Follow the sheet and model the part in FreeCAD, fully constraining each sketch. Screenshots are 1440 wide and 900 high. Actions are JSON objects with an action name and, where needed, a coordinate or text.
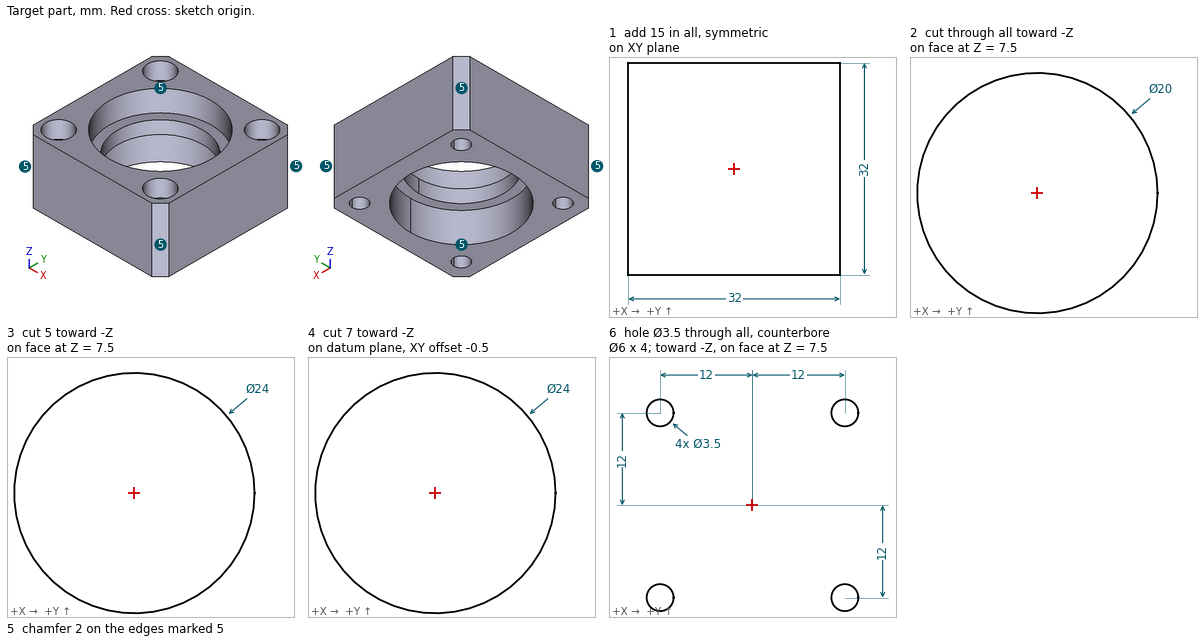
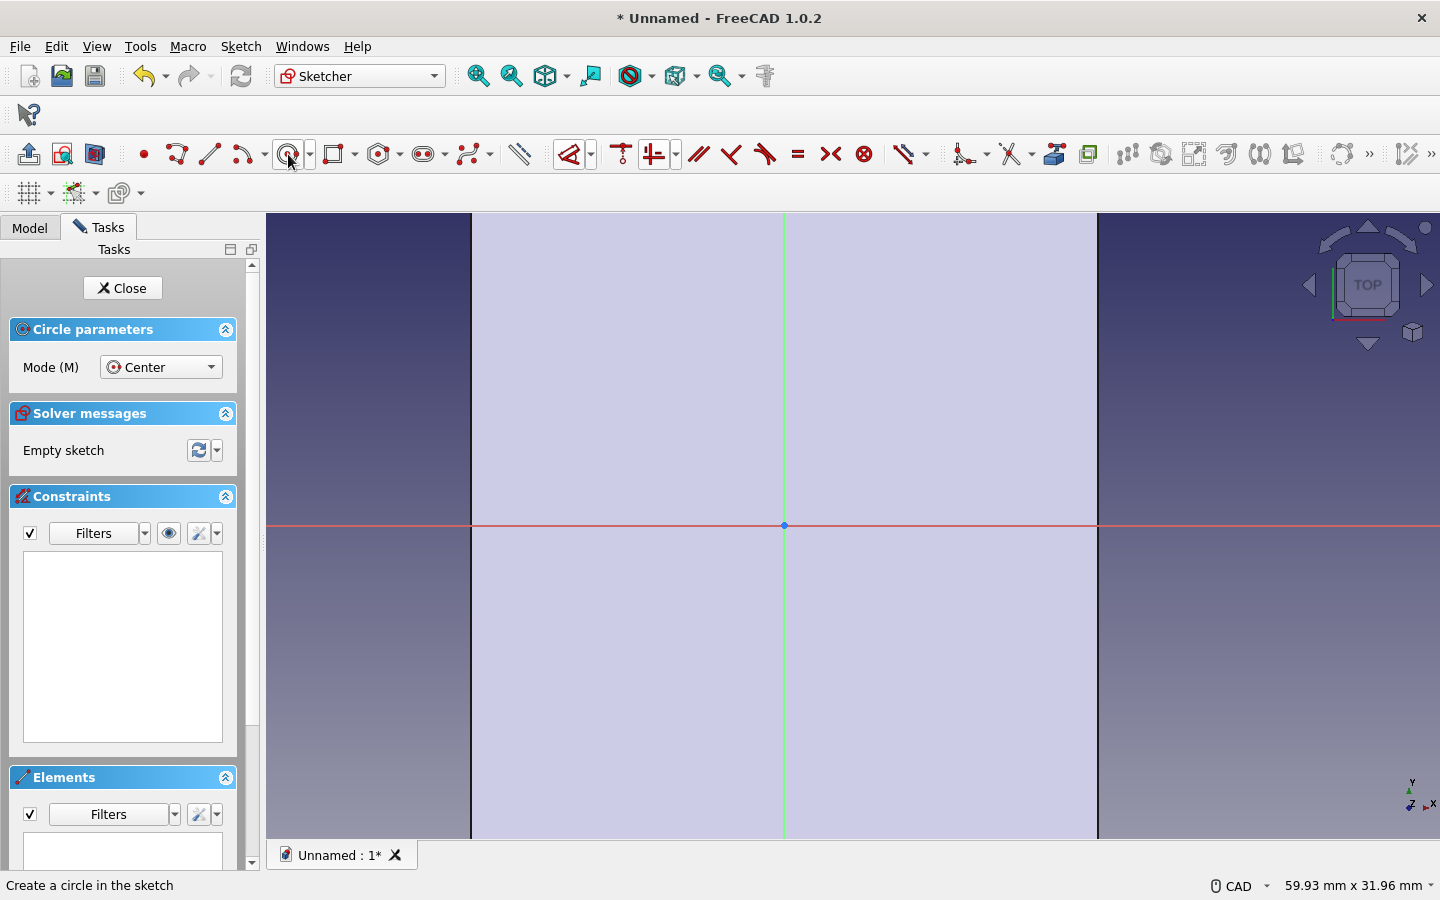
{"action": "left_click", "coordinate": [784, 526]}
{"action": "left_click", "coordinate": [923, 387]}
{"action": "key", "text": "Escape"}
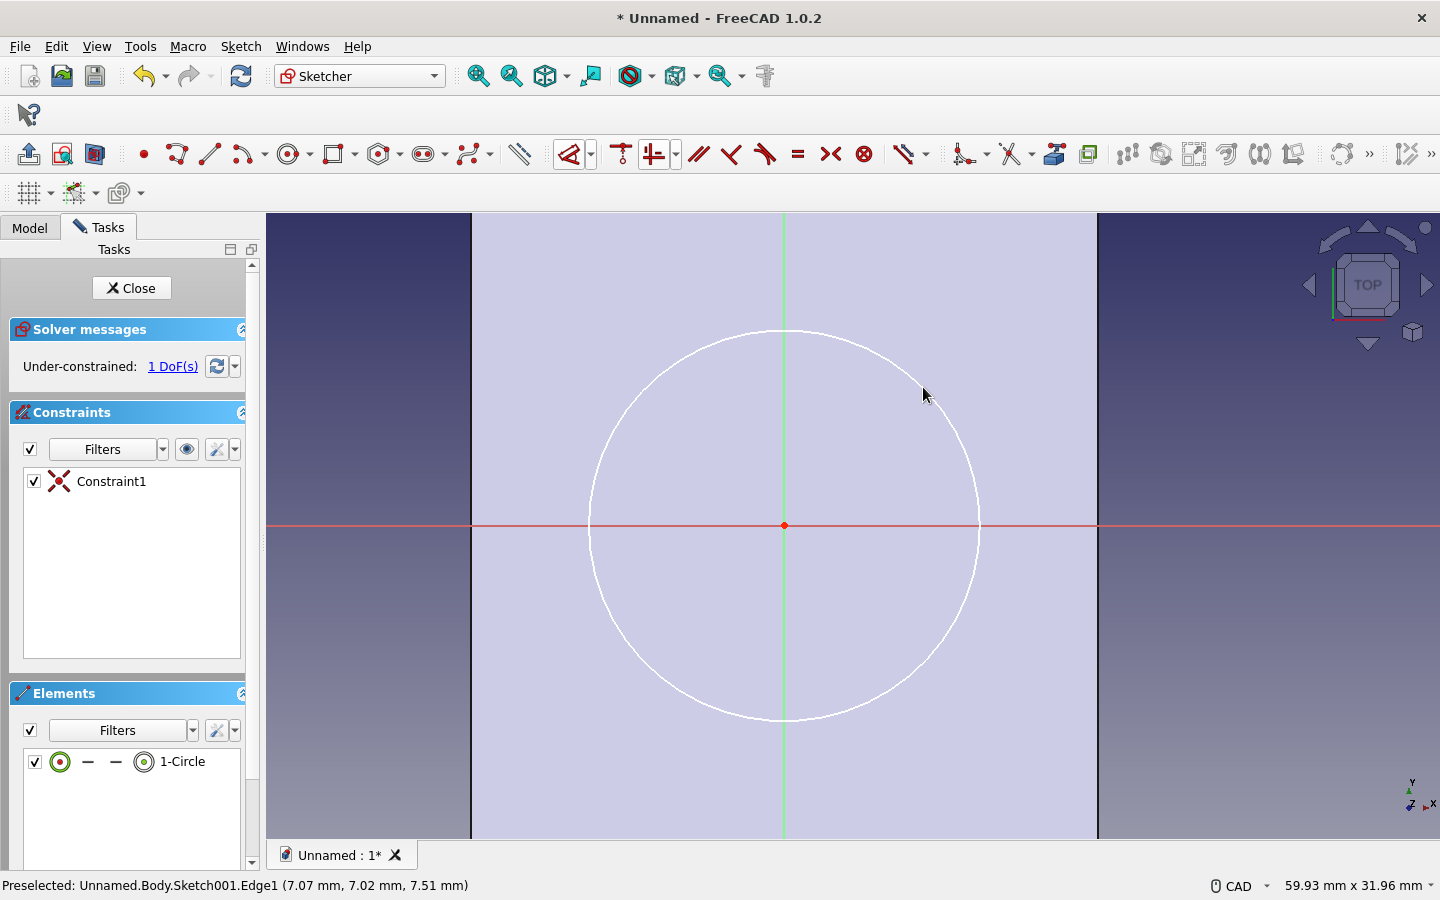
{"action": "left_click", "coordinate": [922, 387]}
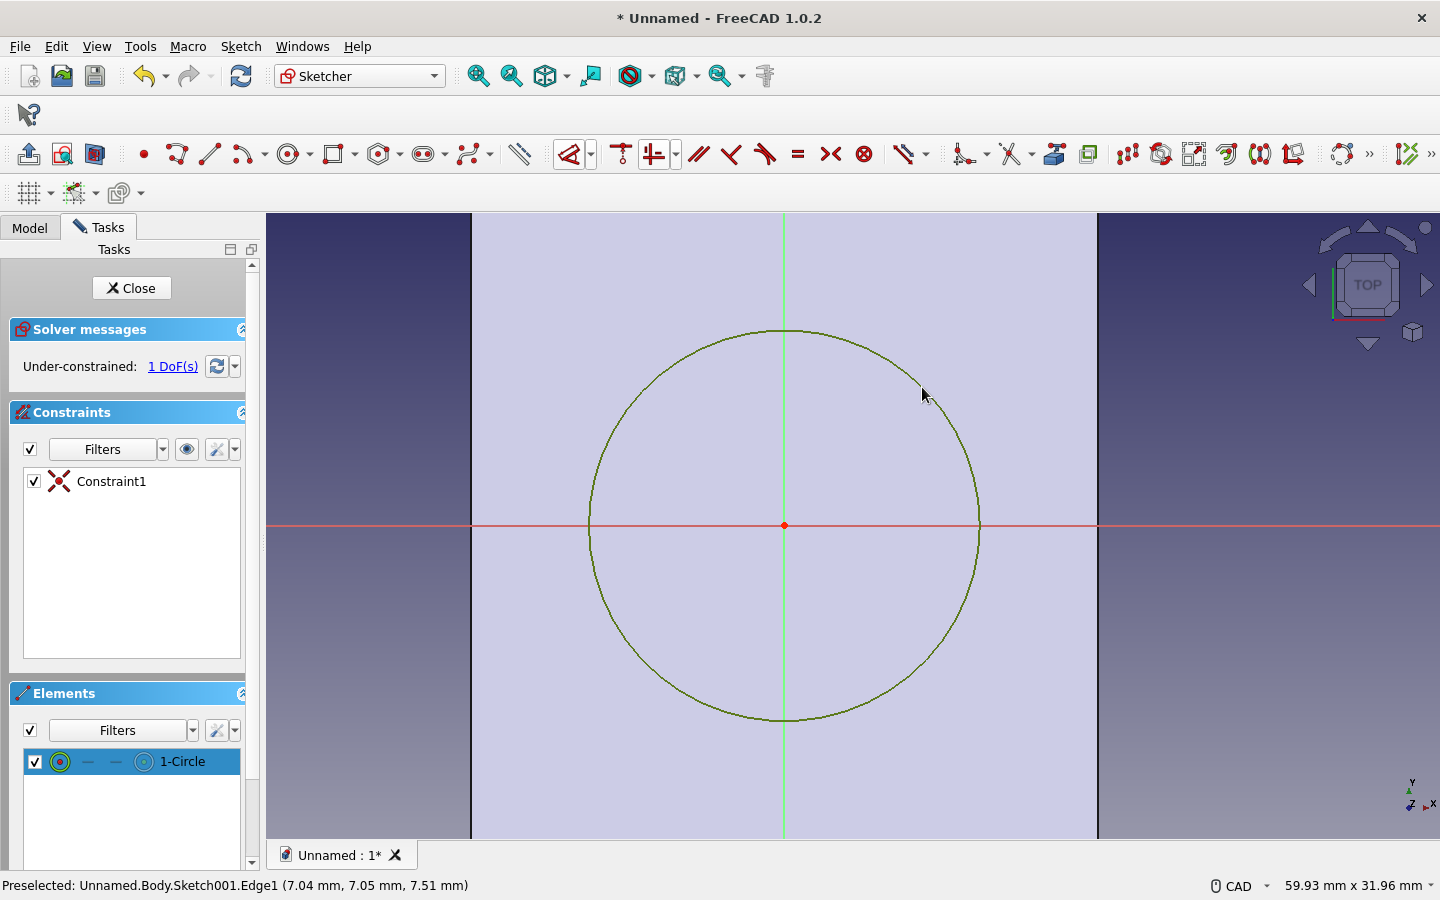
{"action": "left_click", "coordinate": [590, 154]}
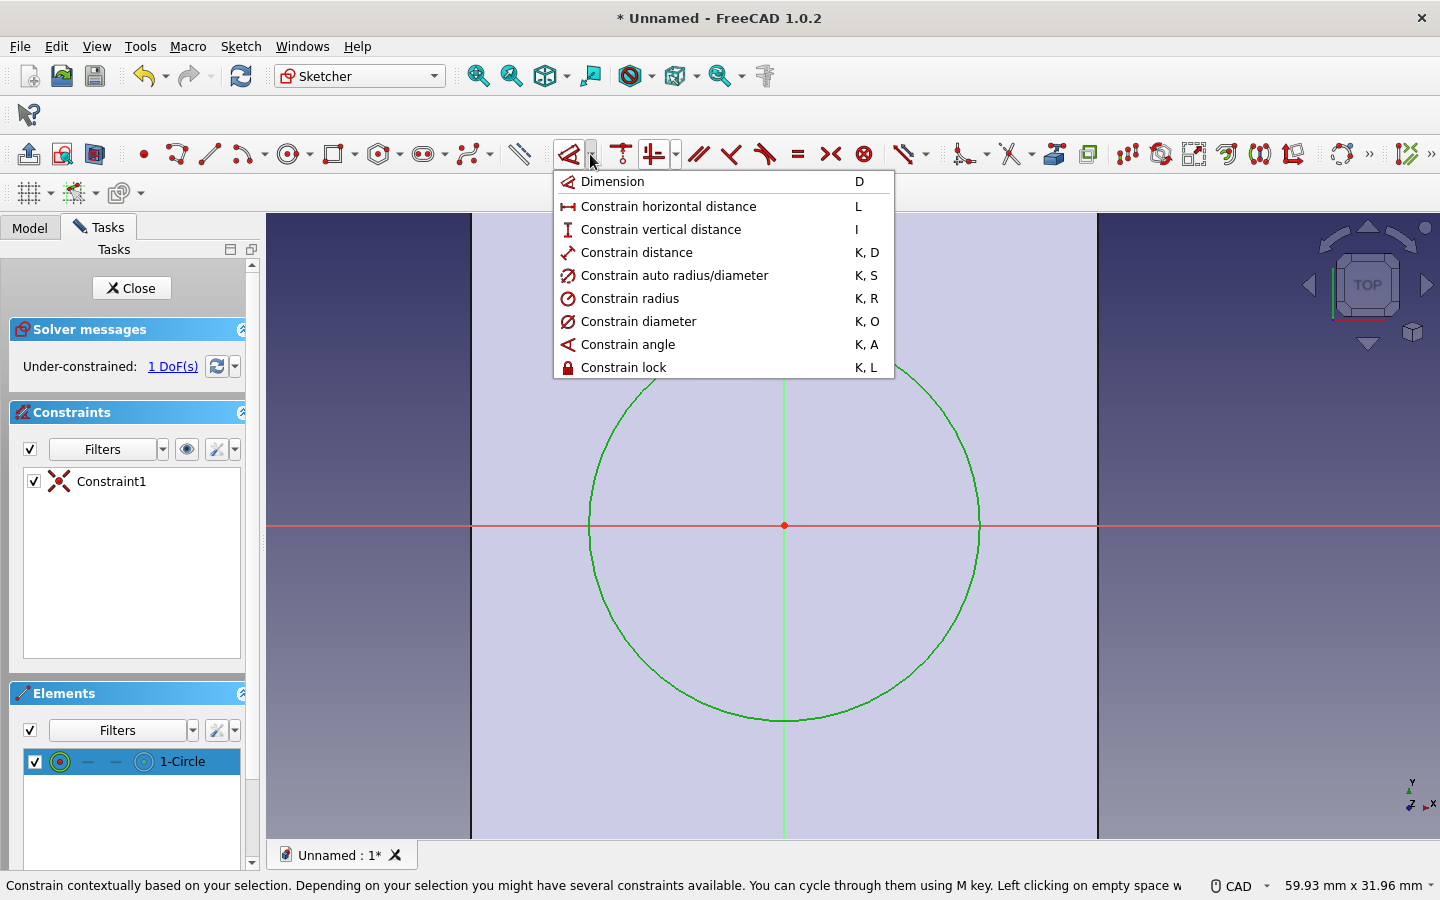
{"action": "left_click", "coordinate": [724, 322]}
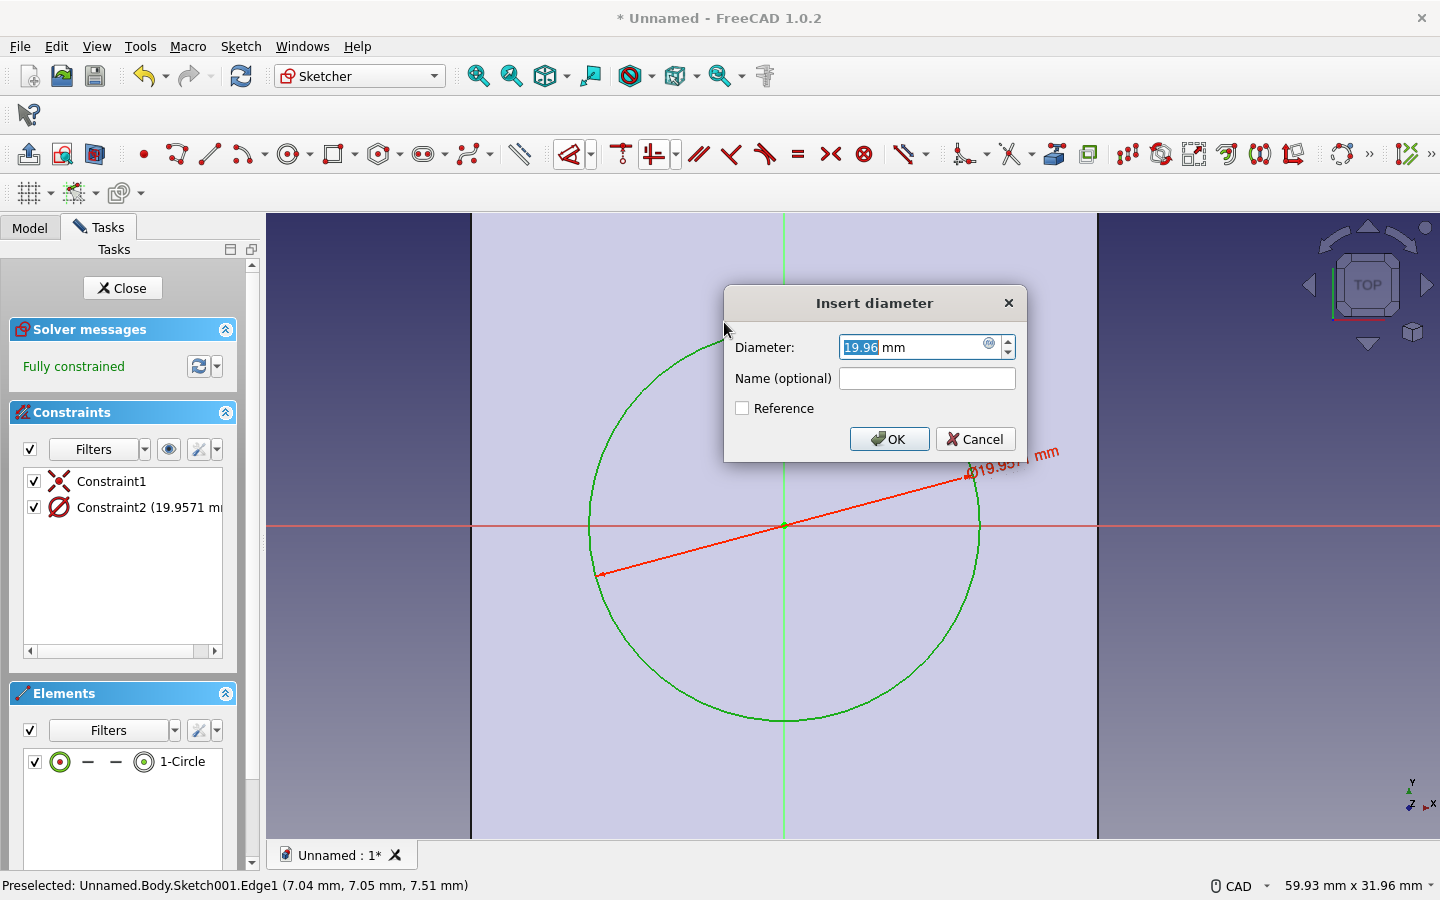
{"action": "type", "text": "20"}
{"action": "key", "text": "Return"}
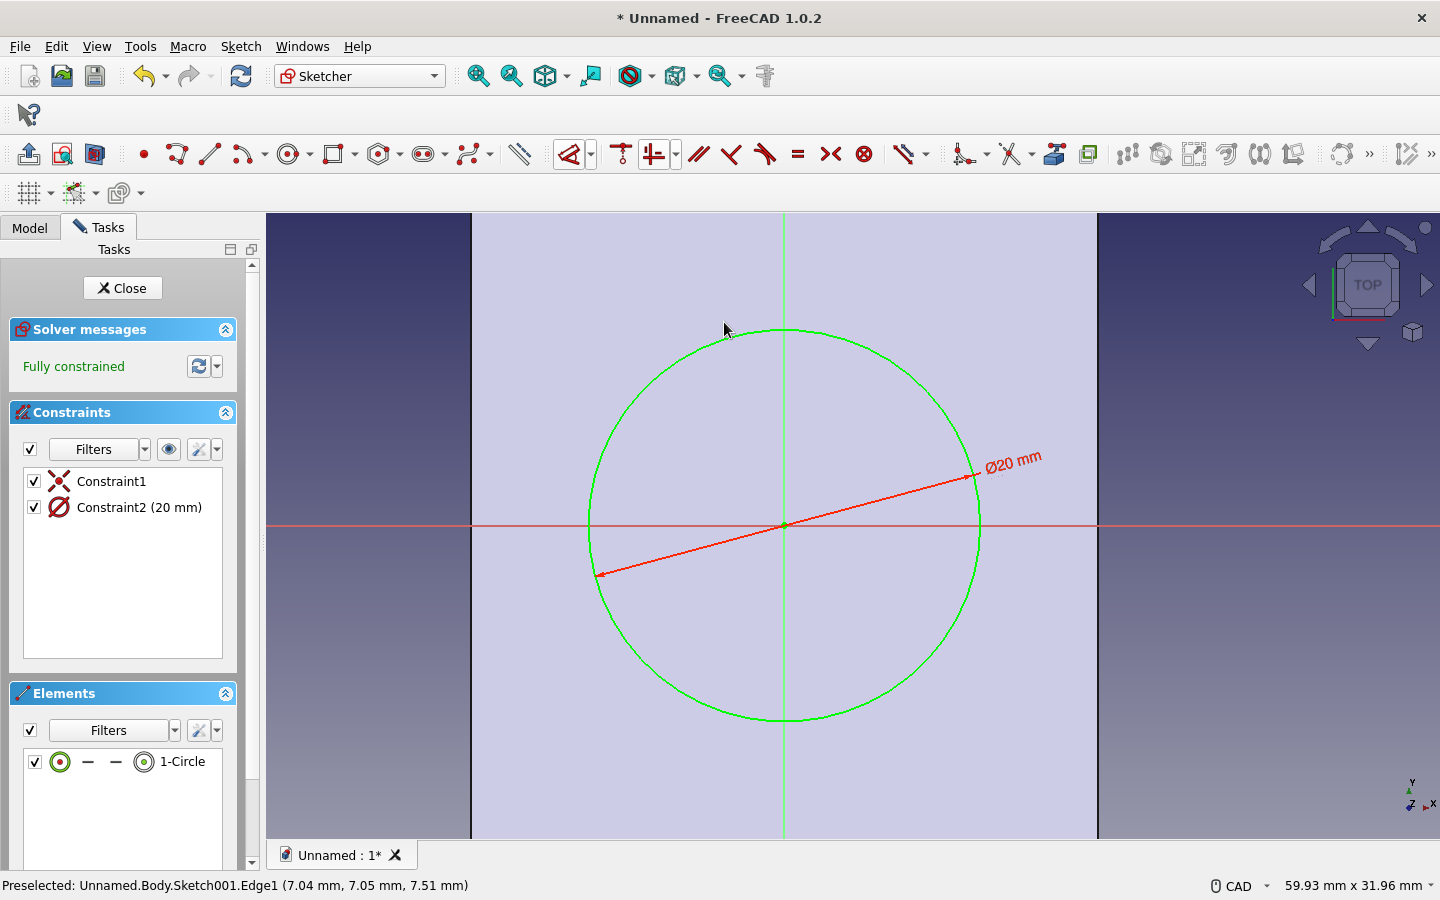
{"action": "left_click", "coordinate": [123, 288]}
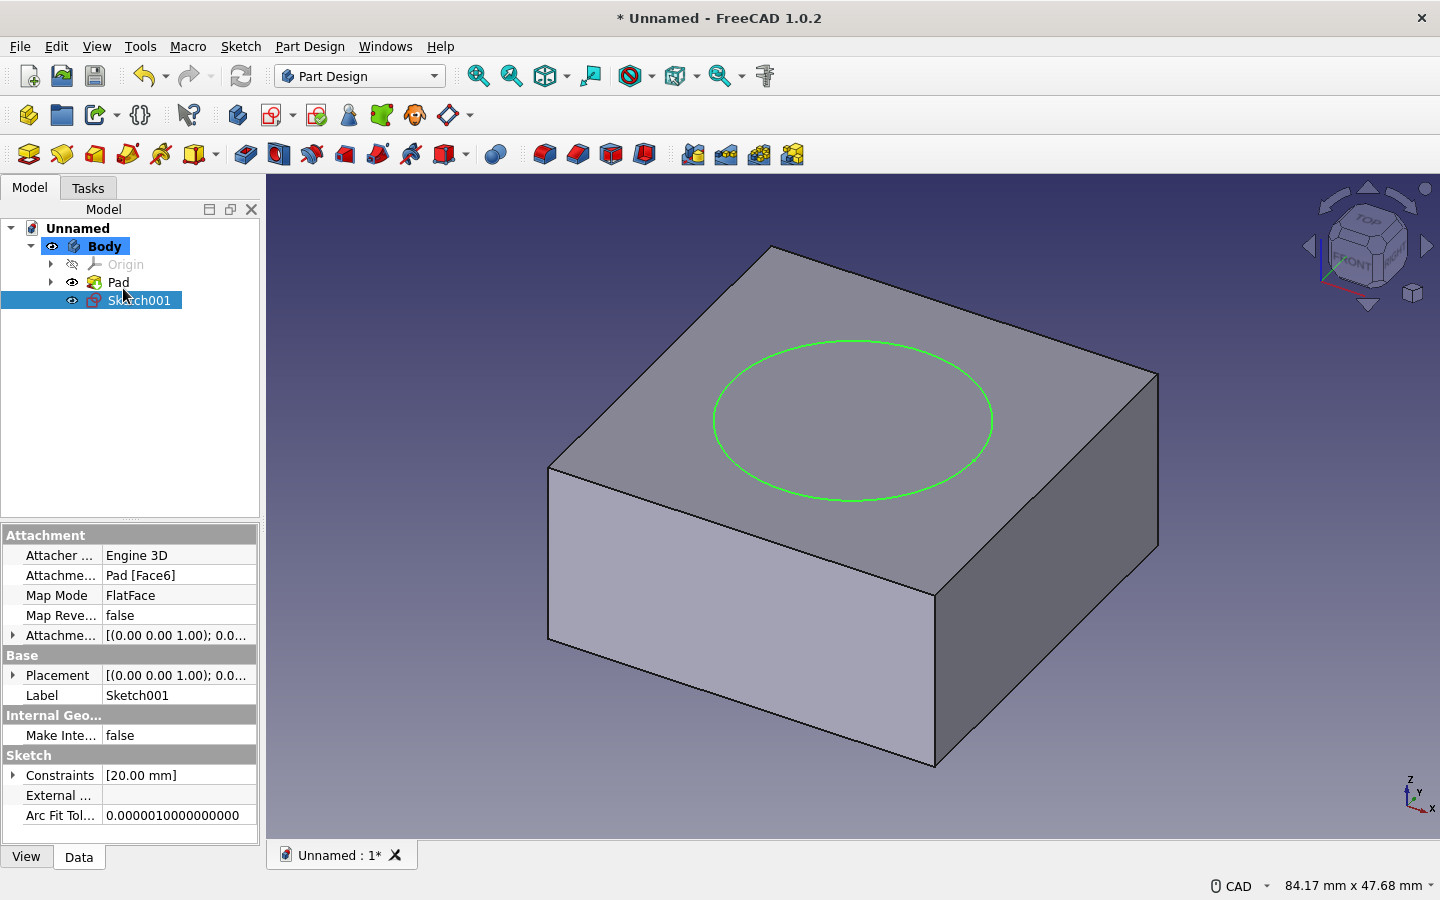
{"action": "left_click", "coordinate": [246, 154]}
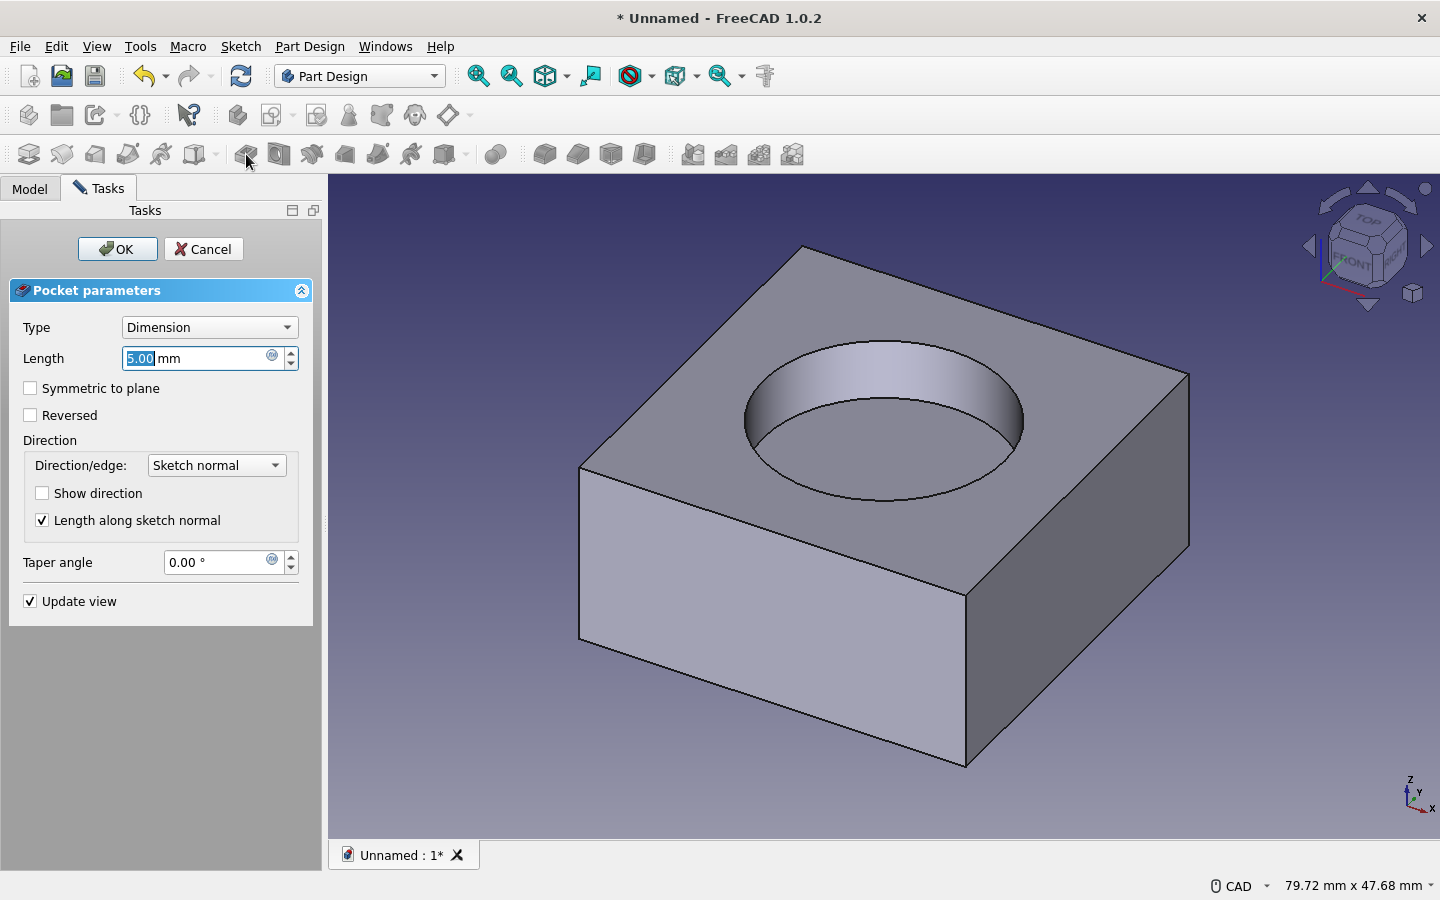
{"action": "left_click", "coordinate": [210, 328]}